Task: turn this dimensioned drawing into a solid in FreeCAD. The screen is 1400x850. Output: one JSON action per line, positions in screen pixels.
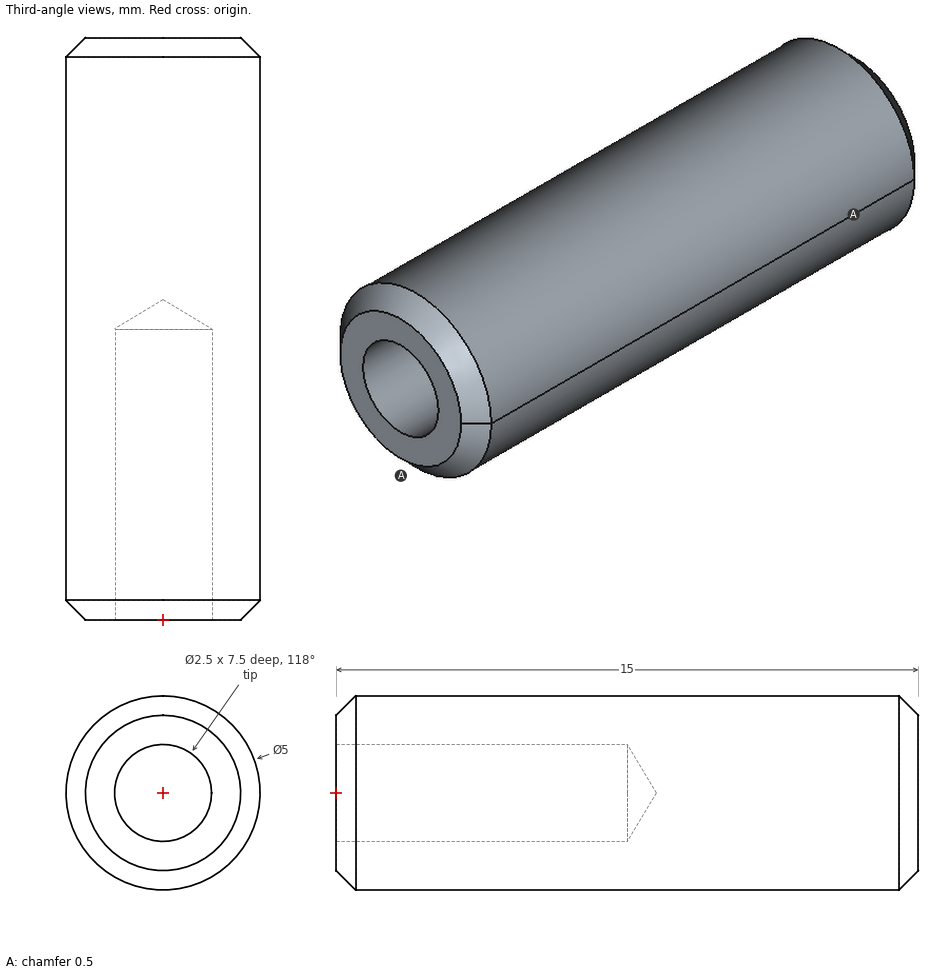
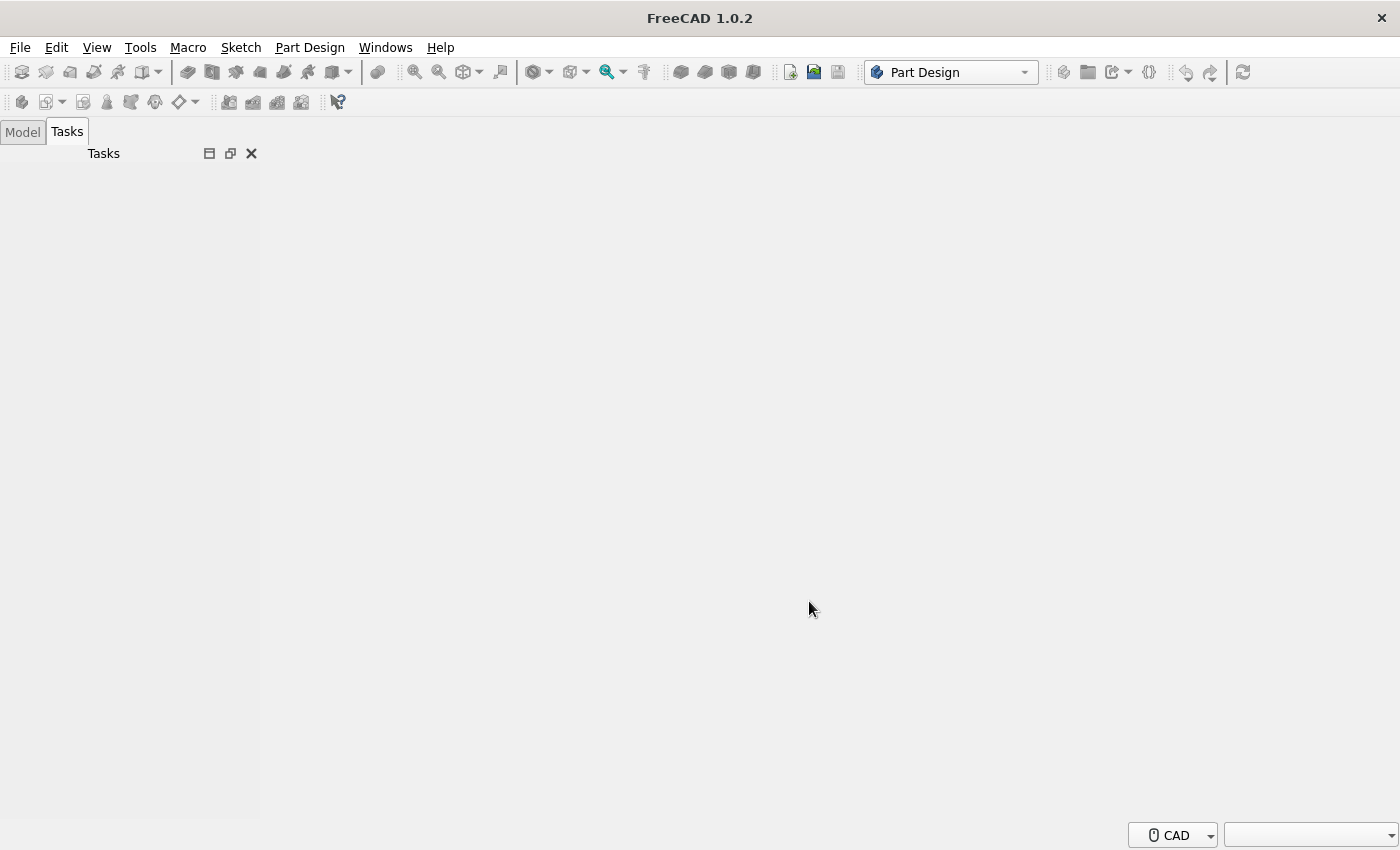
{"action": "left_click", "coordinate": [790, 72]}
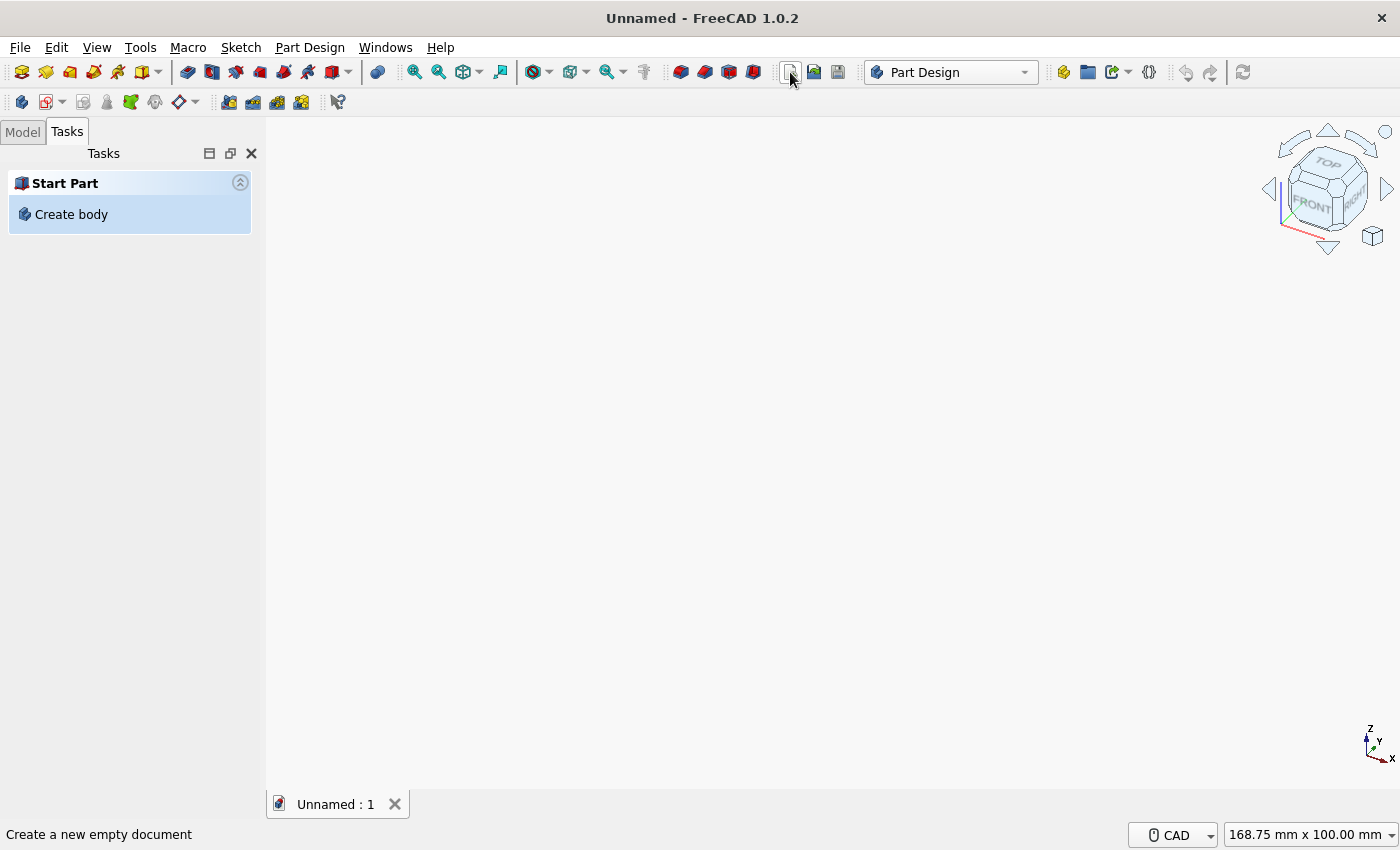
{"action": "left_click", "coordinate": [46, 102]}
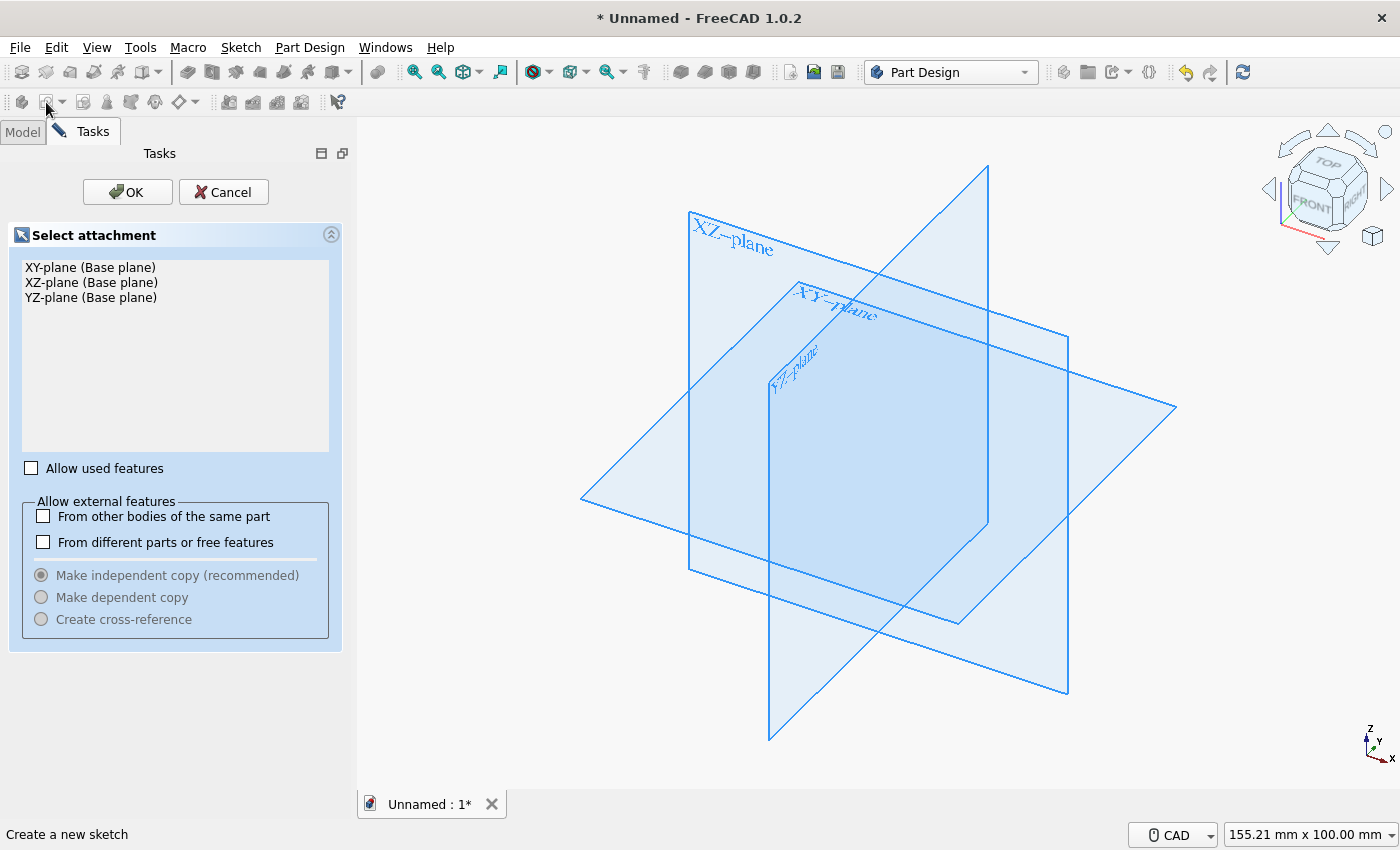
{"action": "left_click", "coordinate": [82, 282]}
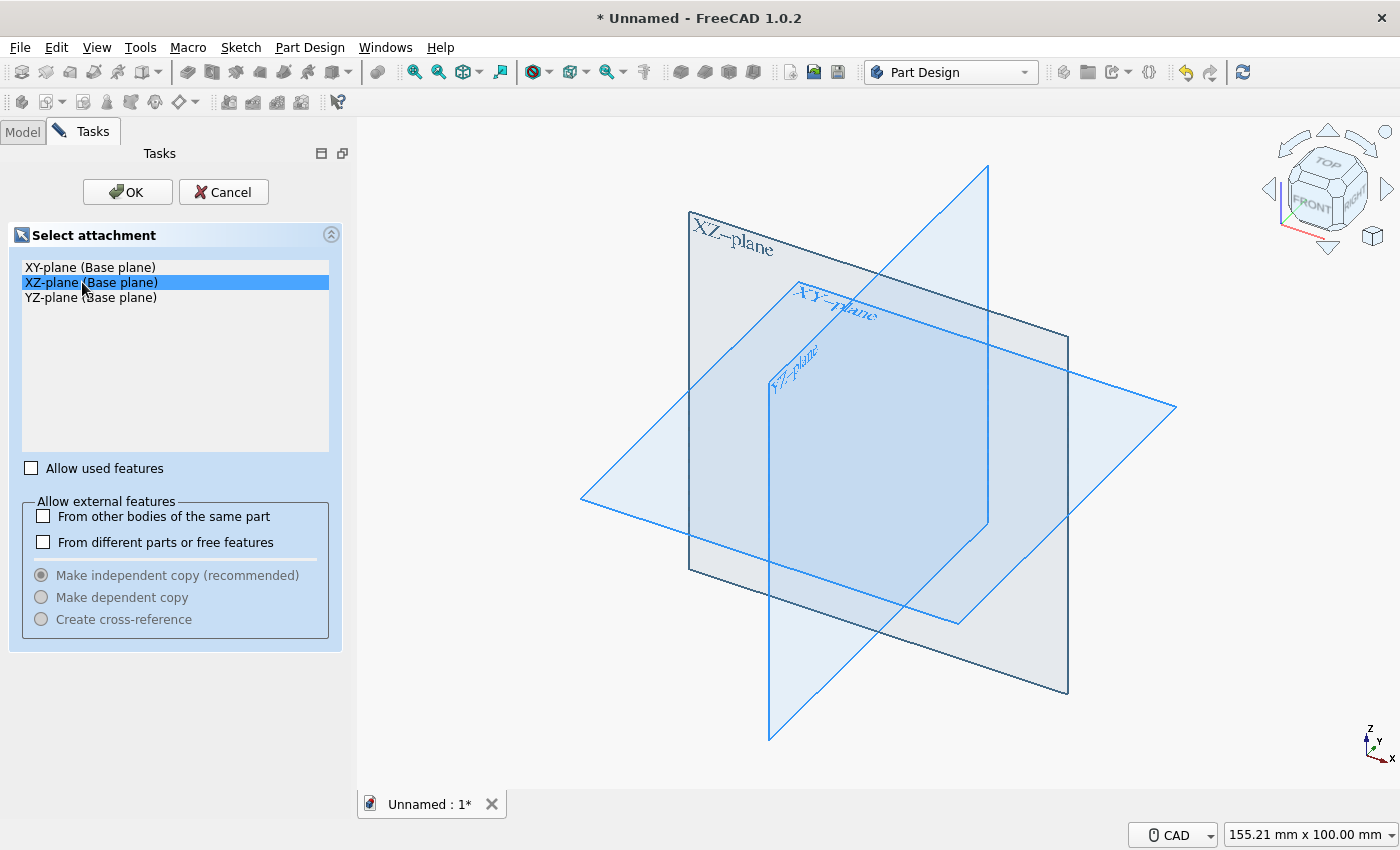
{"action": "left_click", "coordinate": [128, 192]}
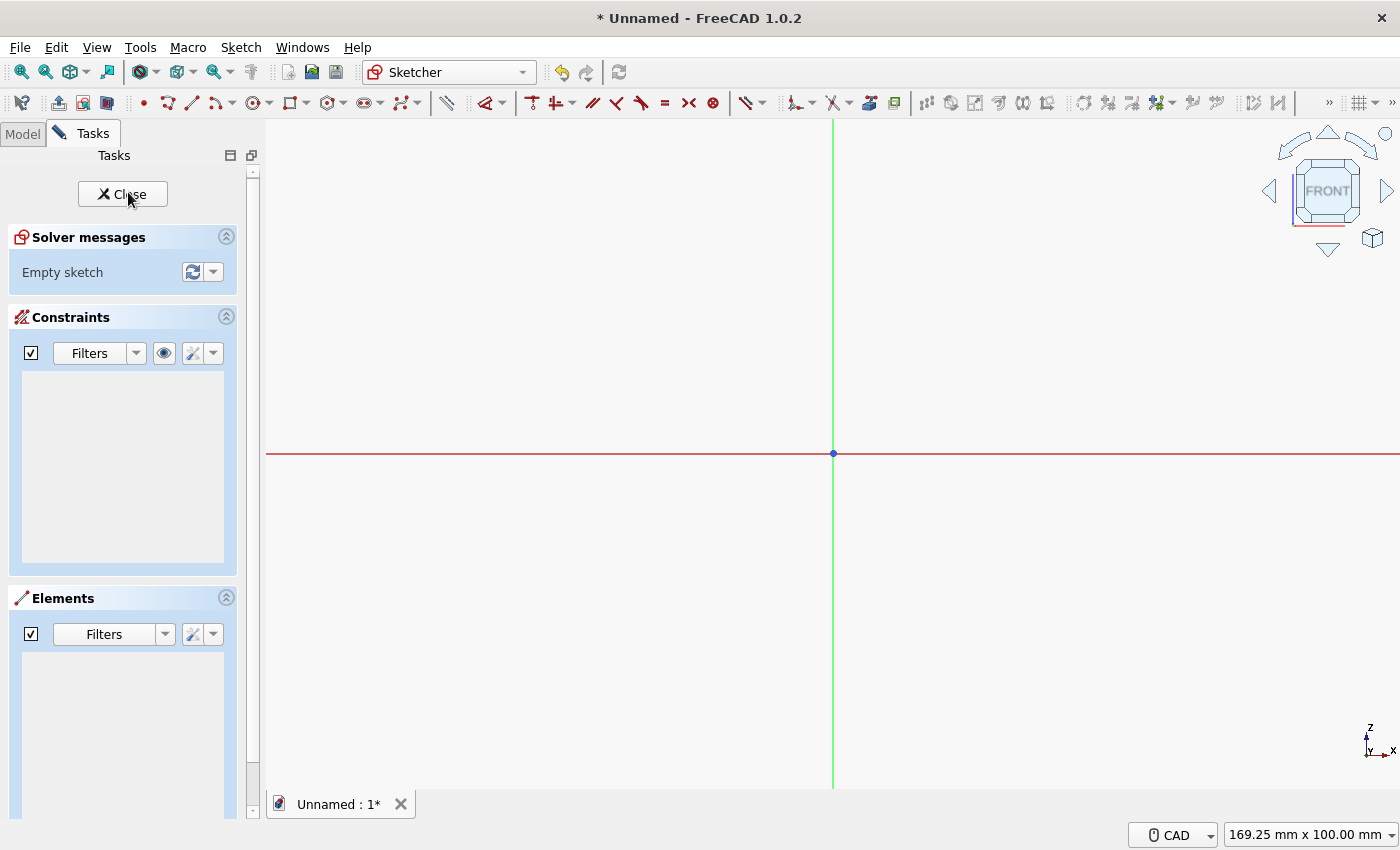
{"action": "scroll", "coordinate": [838, 454], "scroll_direction": "up", "scroll_amount": 13}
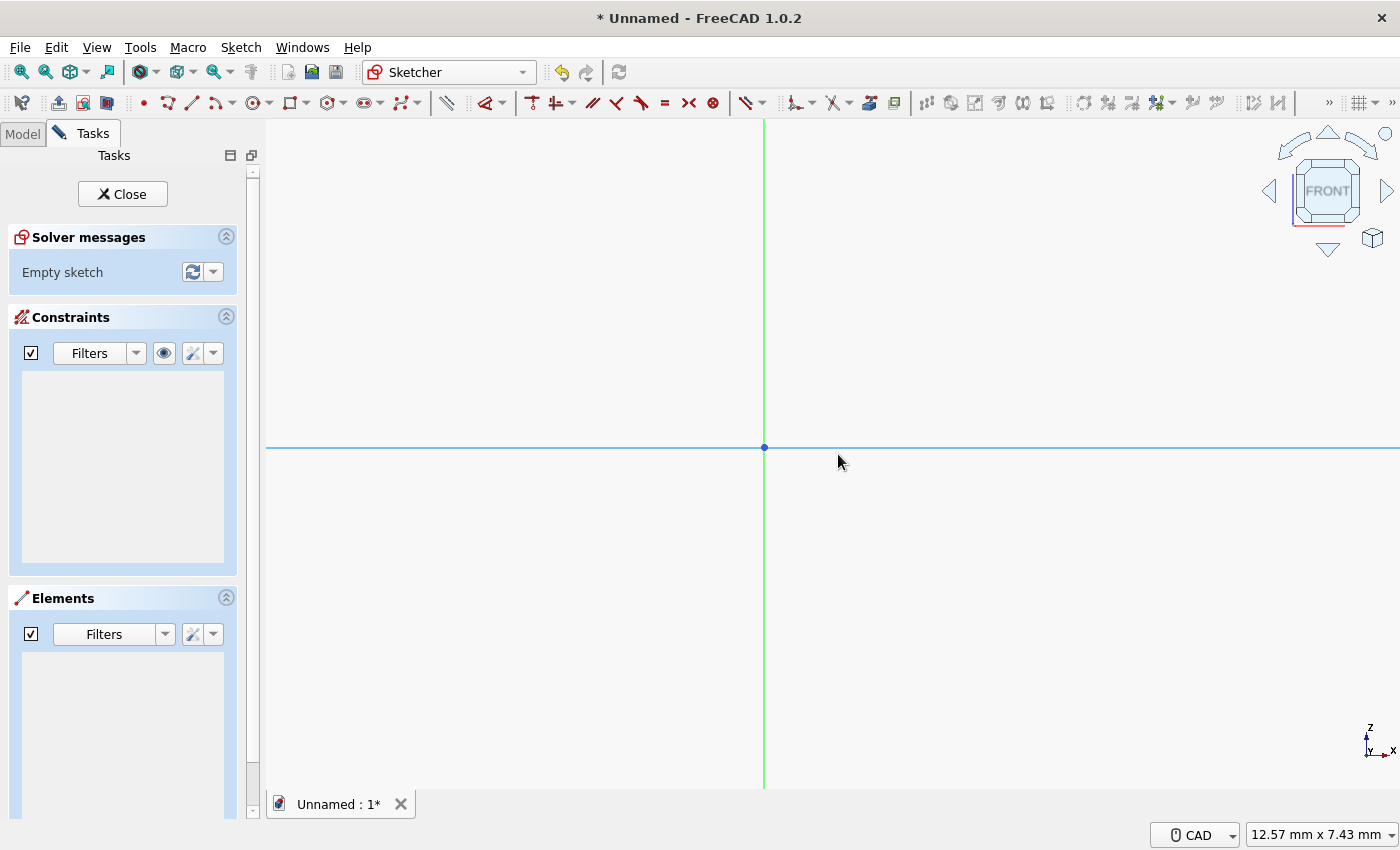
{"action": "left_click", "coordinate": [254, 104]}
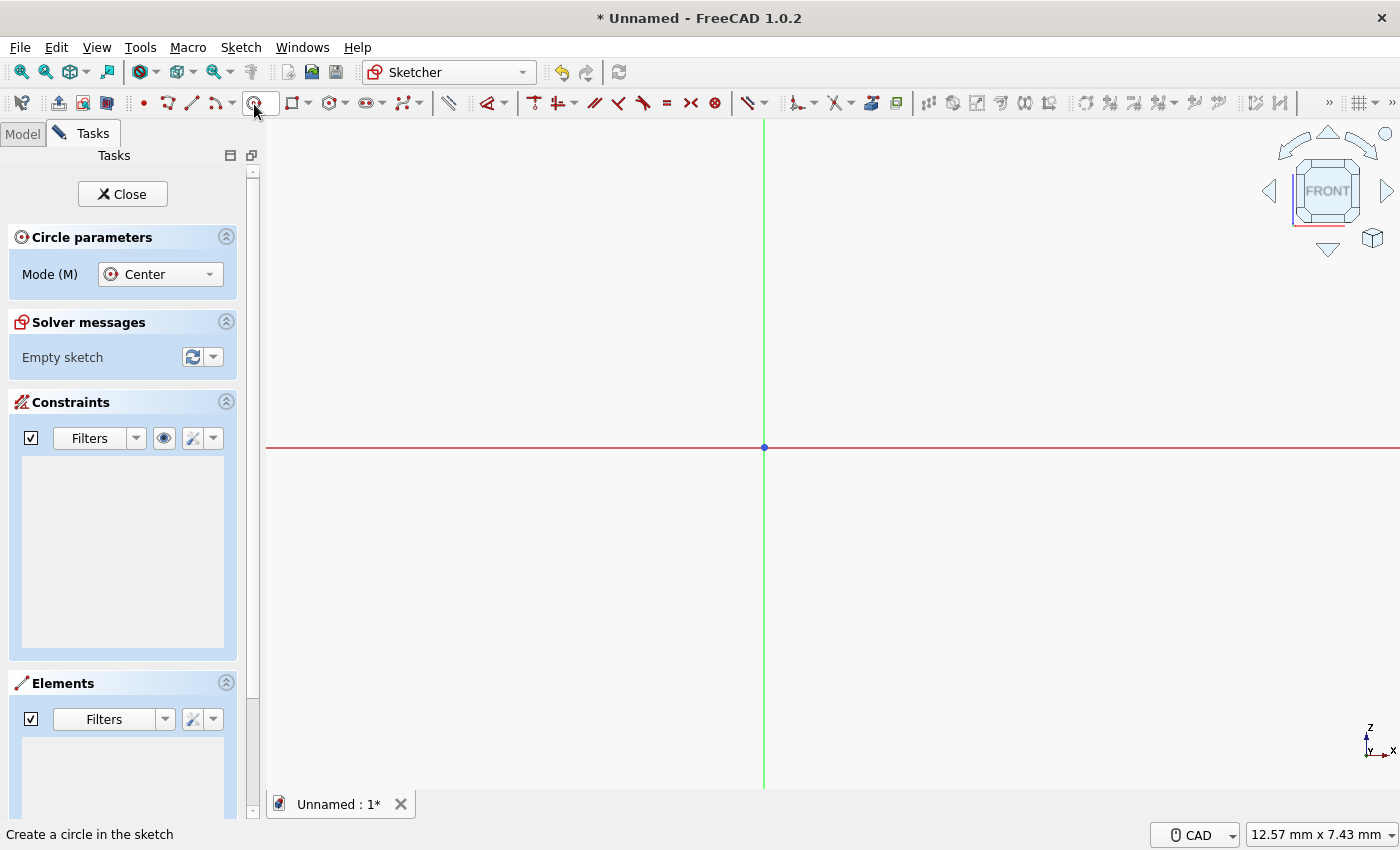
{"action": "left_click", "coordinate": [764, 448]}
{"action": "mouse_move", "coordinate": [924, 288]}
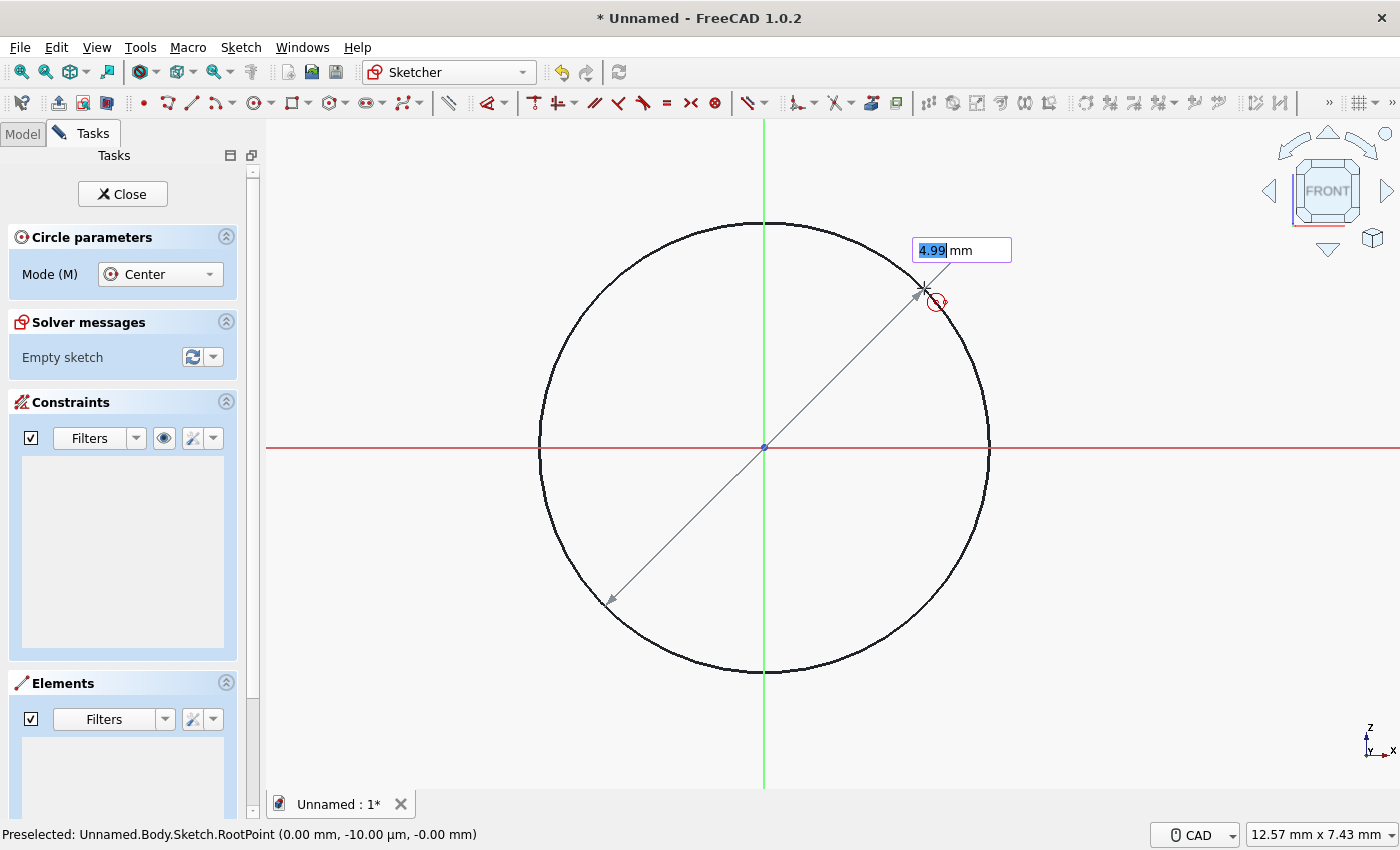
{"action": "type", "text": "5"}
{"action": "key", "text": "Return"}
{"action": "key", "text": "Escape"}